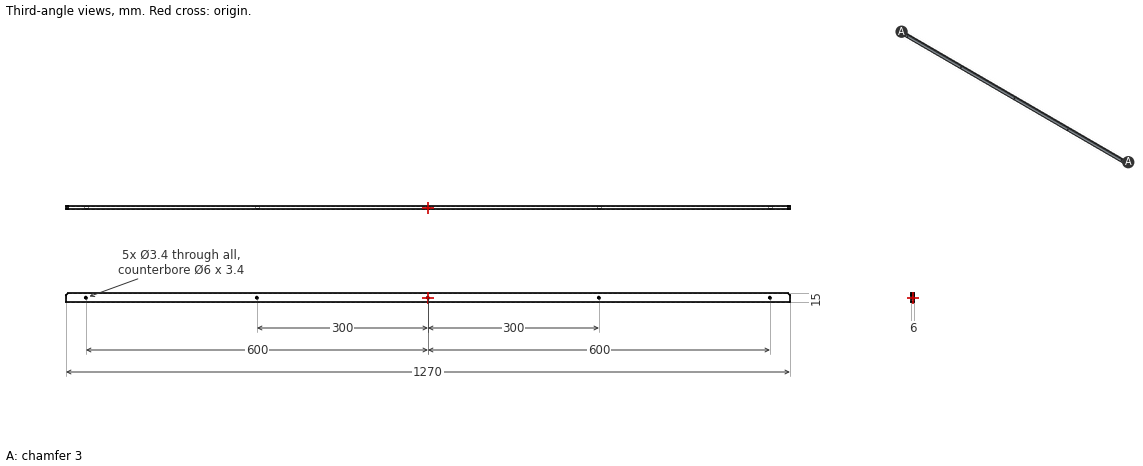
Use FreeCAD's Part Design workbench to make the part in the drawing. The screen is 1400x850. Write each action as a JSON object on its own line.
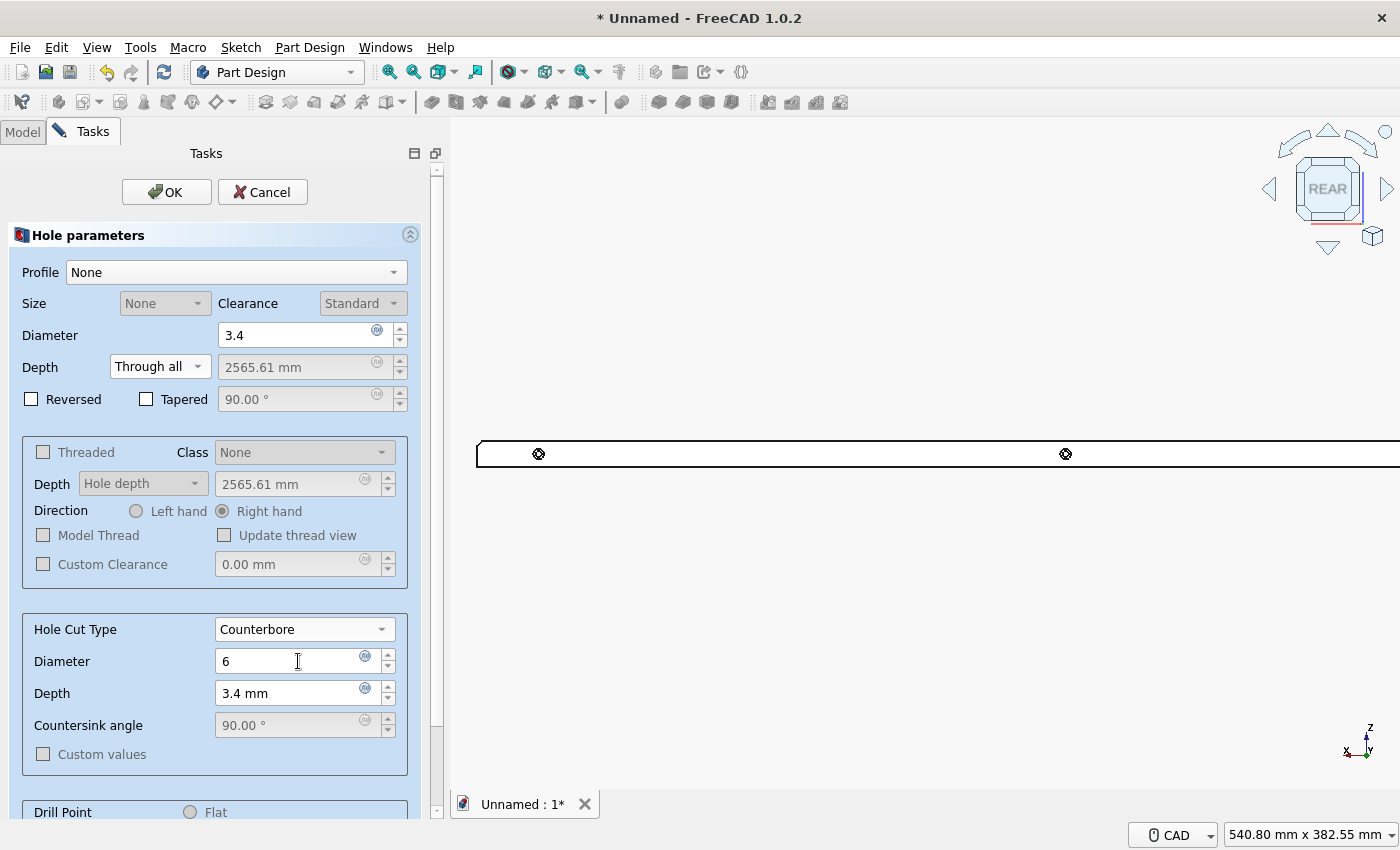
{"action": "left_click", "coordinate": [167, 192]}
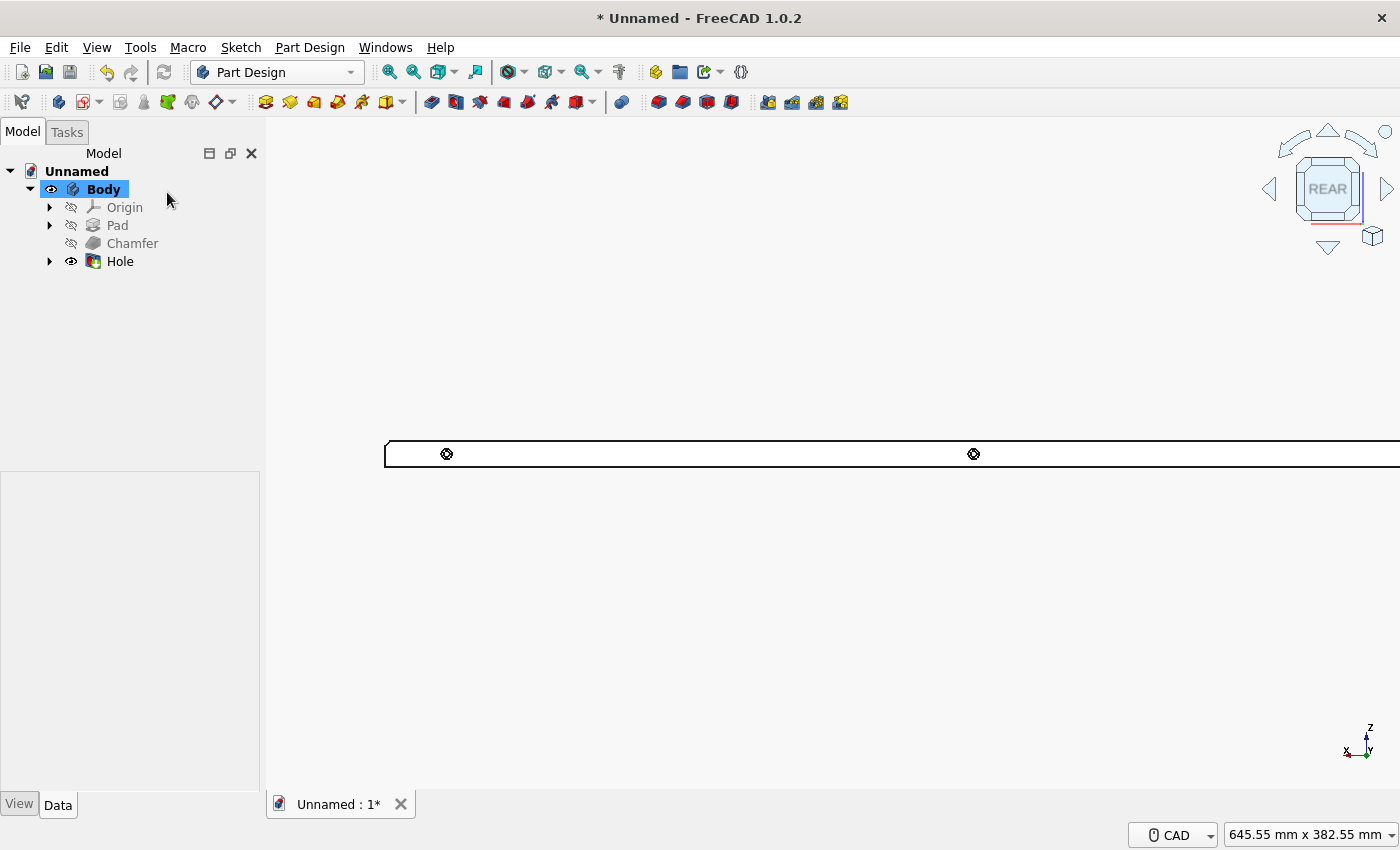
{"action": "key", "text": "0"}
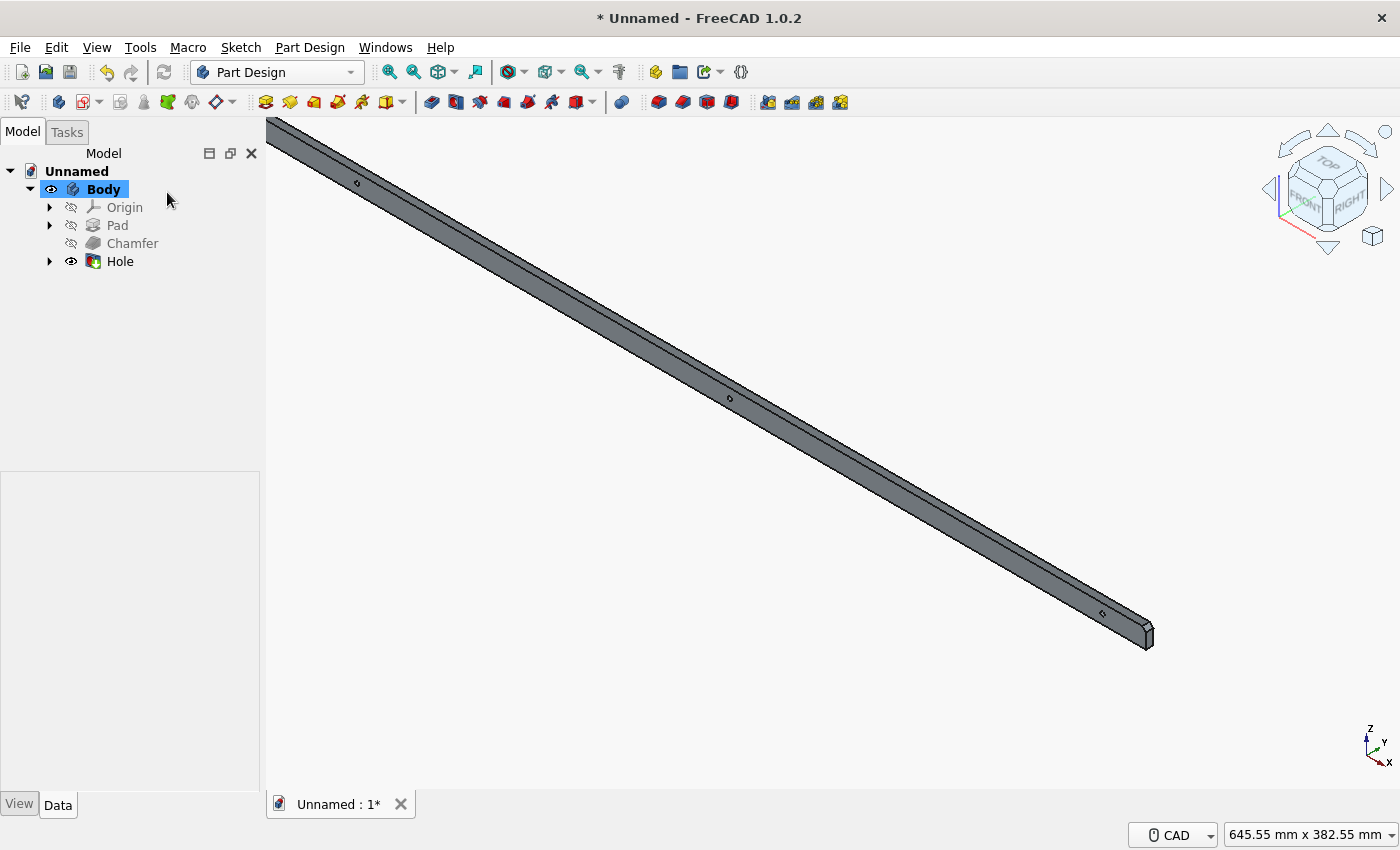
{"action": "key", "text": "v f"}